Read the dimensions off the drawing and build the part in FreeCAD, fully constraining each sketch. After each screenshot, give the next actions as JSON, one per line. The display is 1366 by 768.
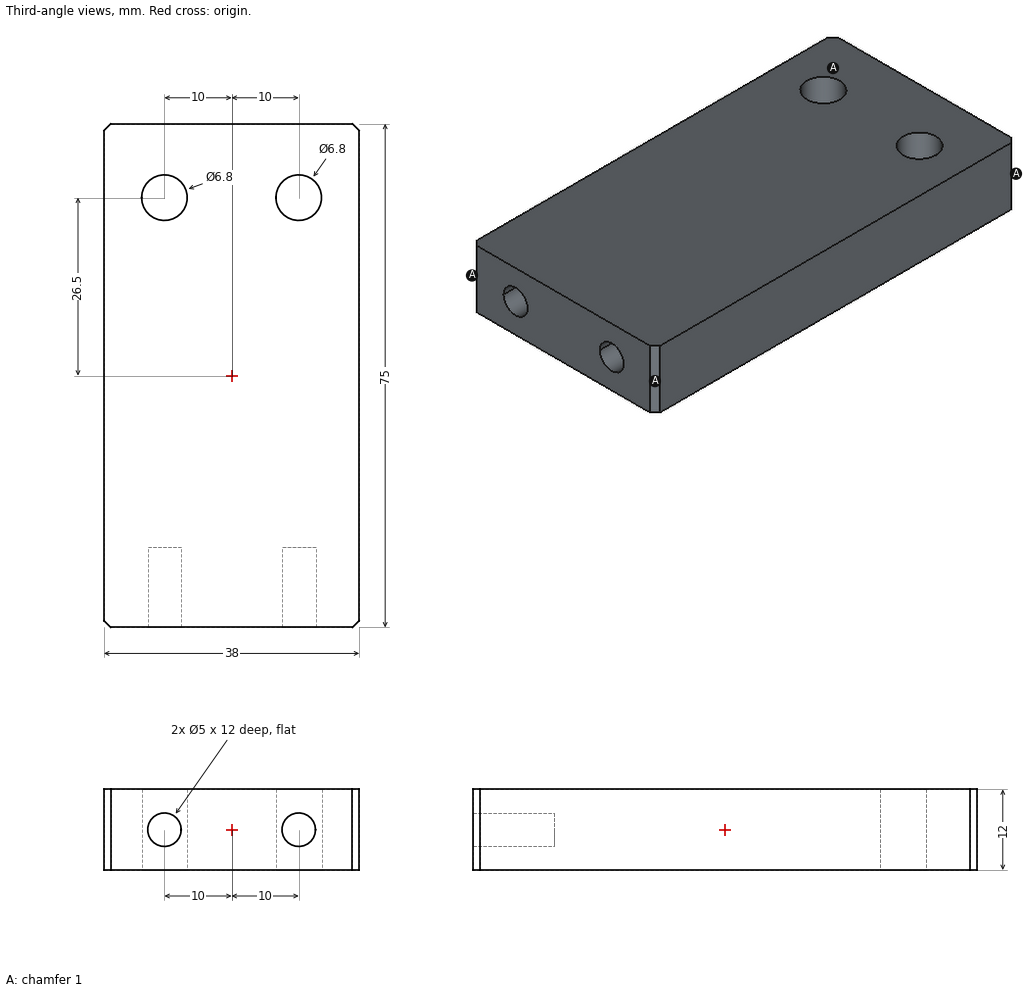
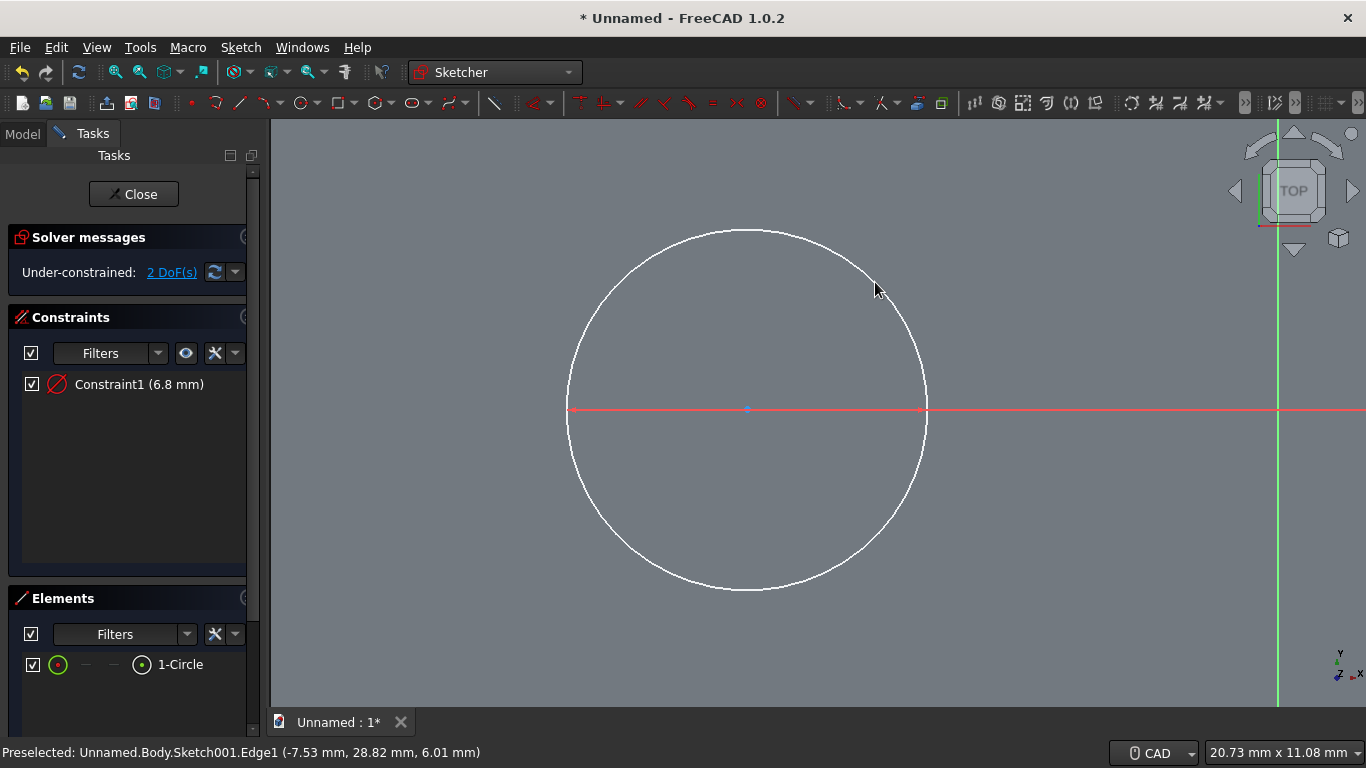
{"action": "key", "text": "d"}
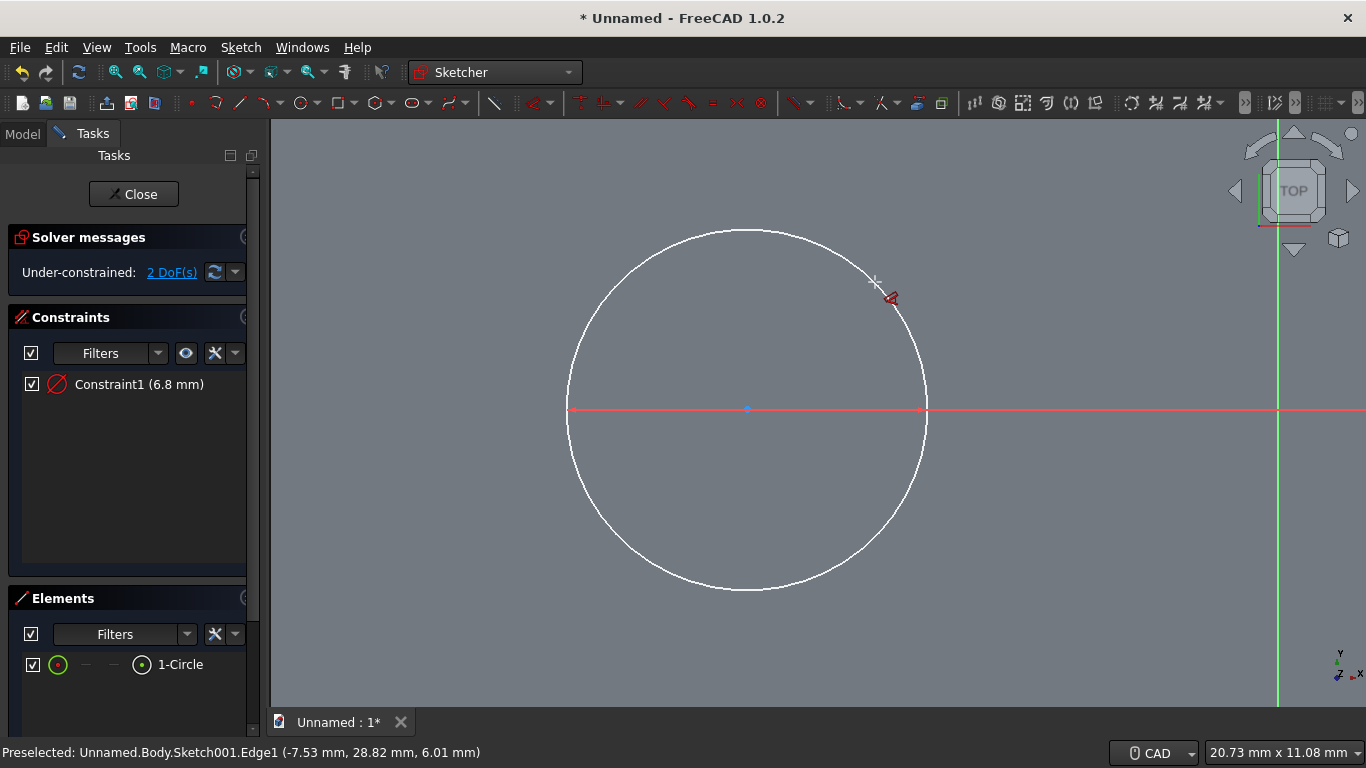
{"action": "left_click", "coordinate": [747, 410]}
{"action": "left_click", "coordinate": [974, 376]}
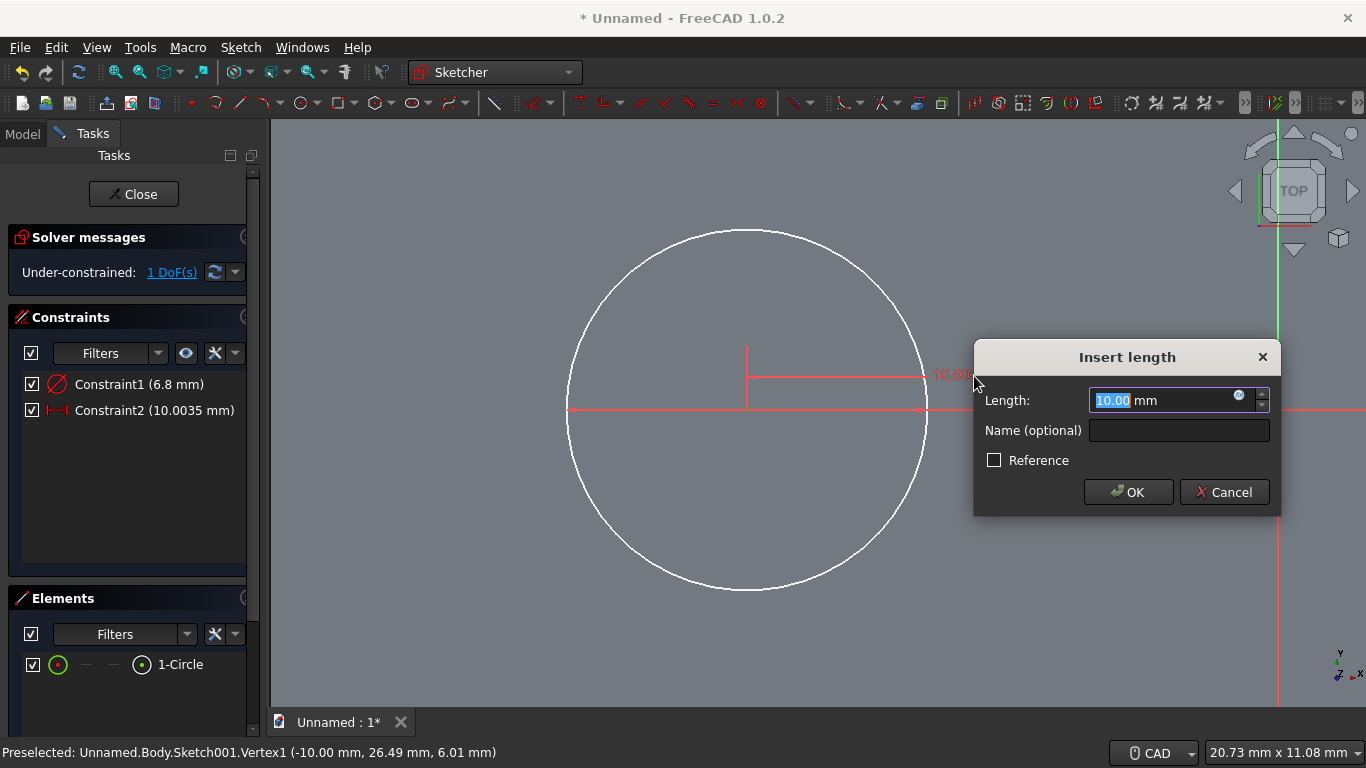
{"action": "type", "text": "10"}
{"action": "key", "text": "Return"}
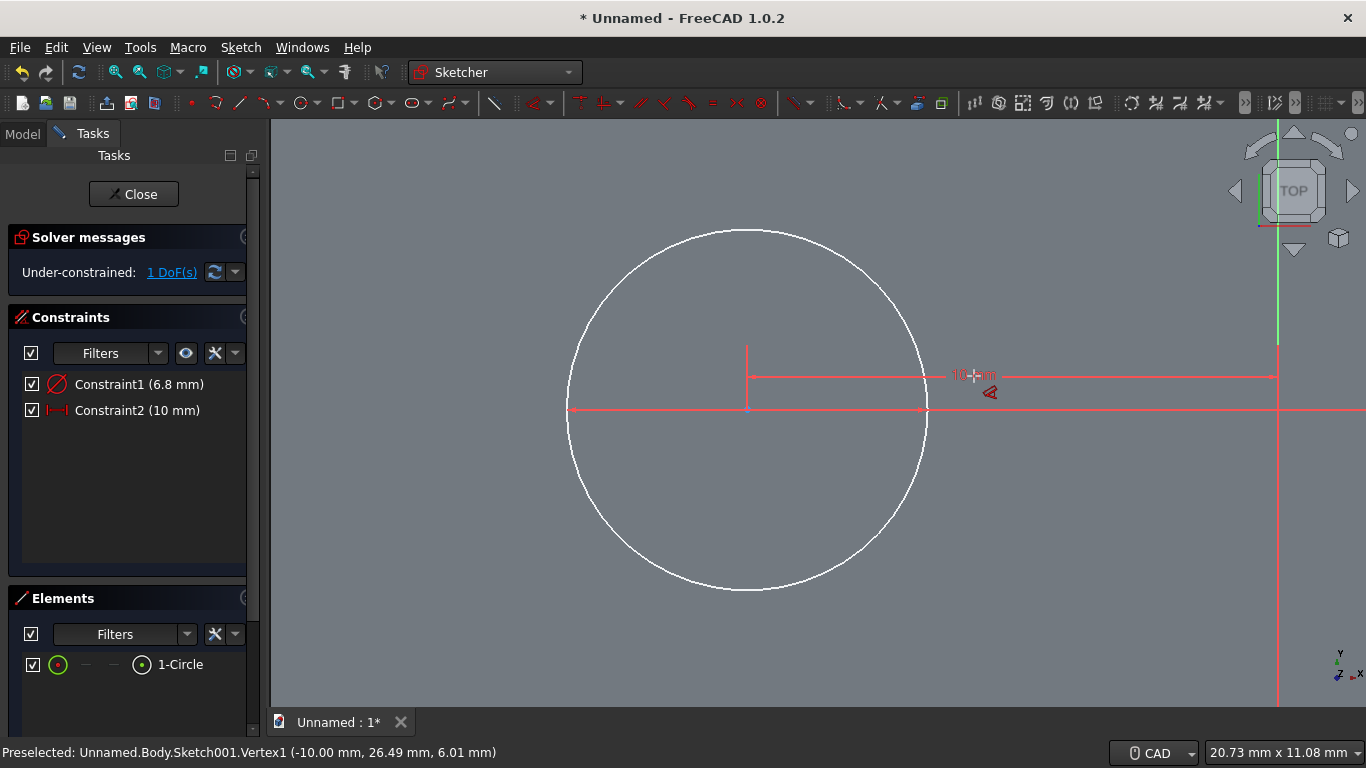
{"action": "left_click", "coordinate": [747, 410]}
{"action": "left_click", "coordinate": [713, 545]}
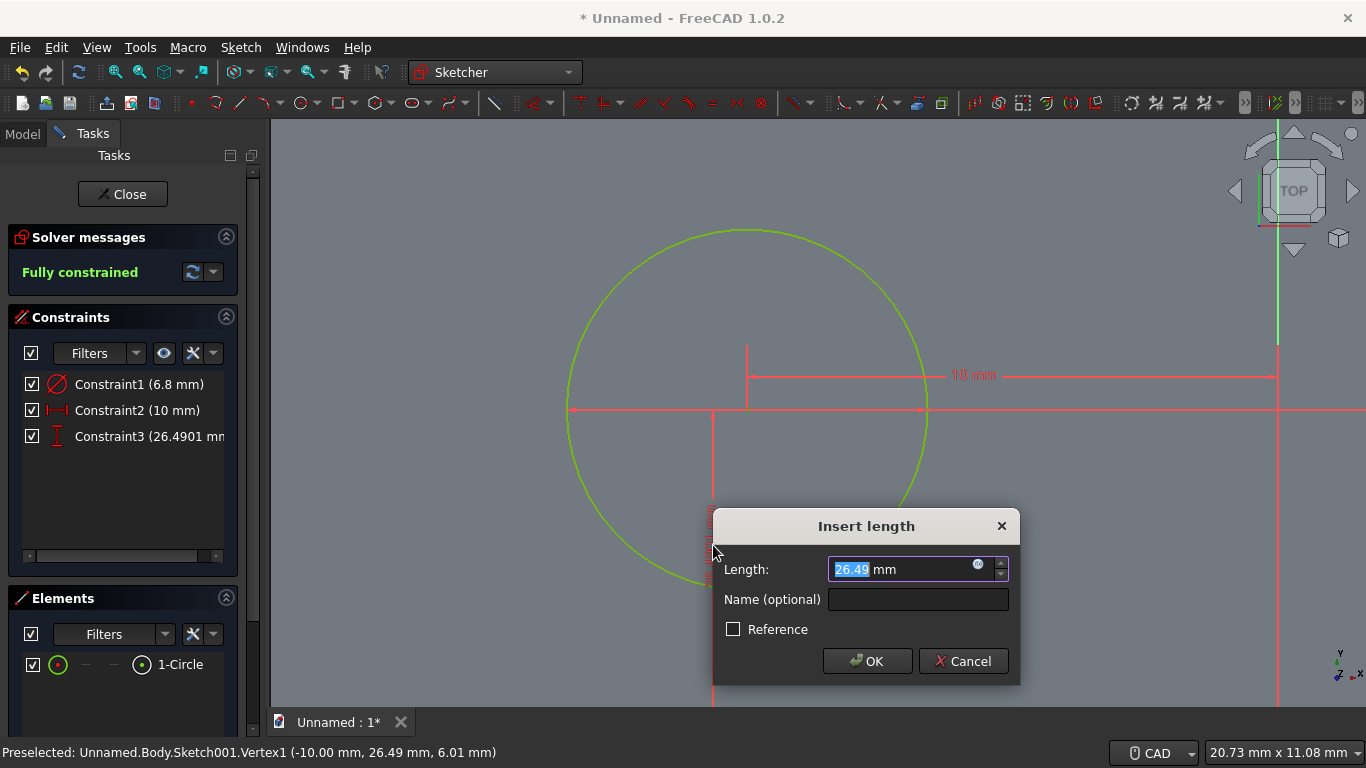
{"action": "type", "text": "26.5"}
{"action": "key", "text": "Return"}
{"action": "key", "text": "Escape"}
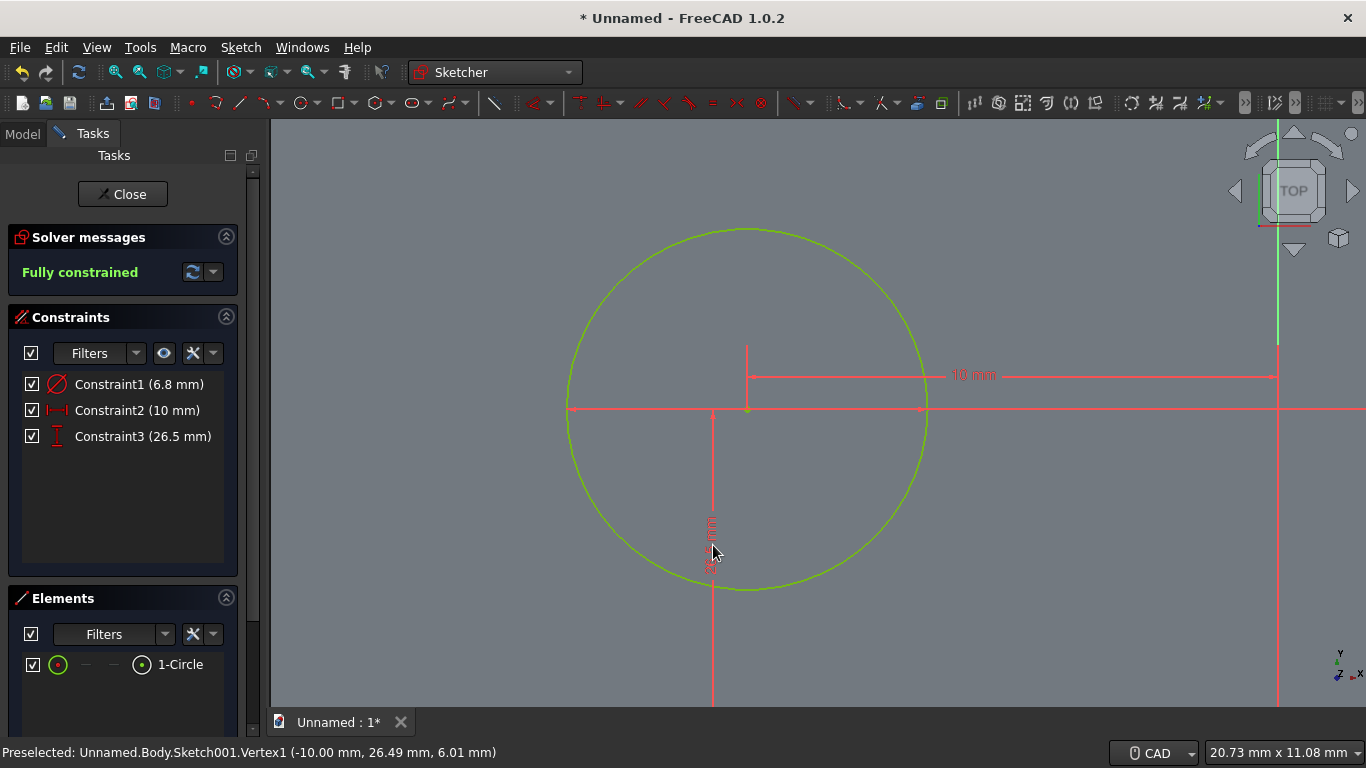
{"action": "left_click", "coordinate": [123, 194]}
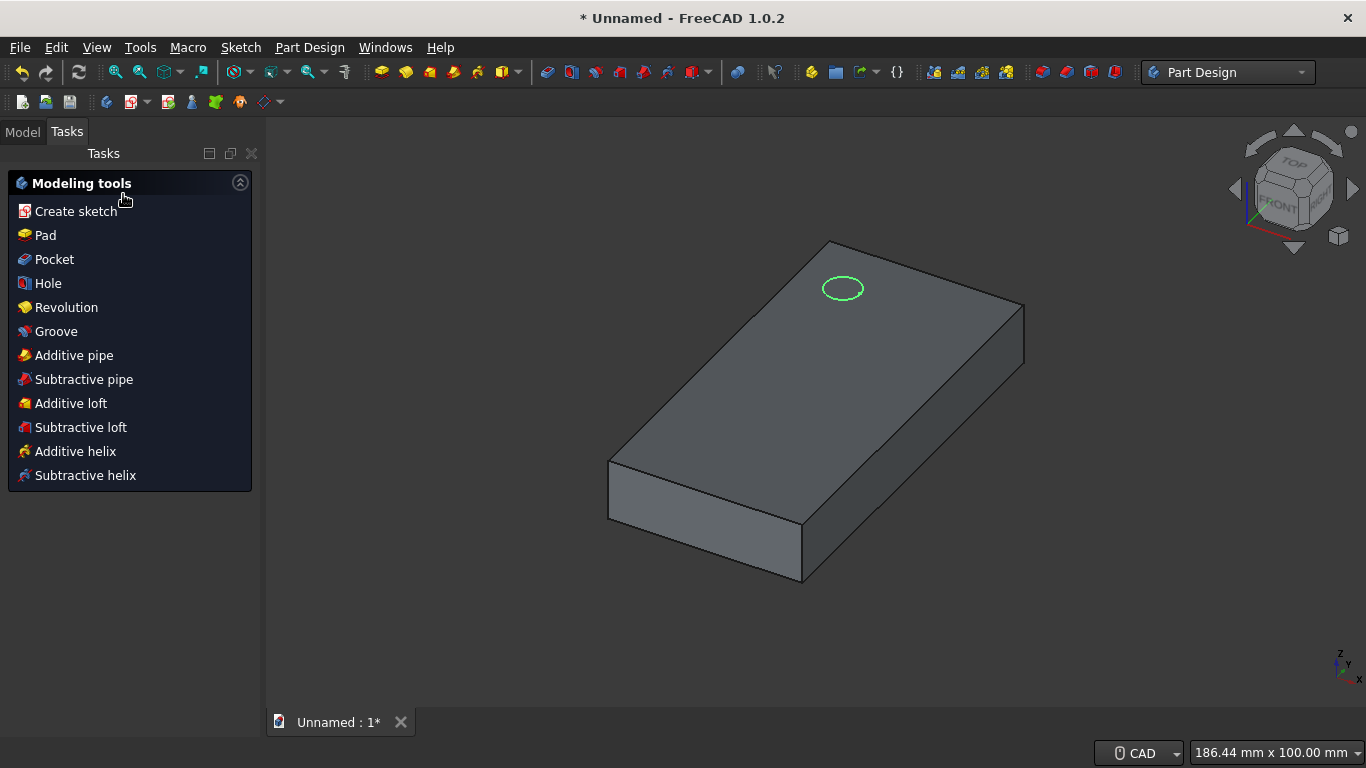
{"action": "left_click", "coordinate": [548, 72]}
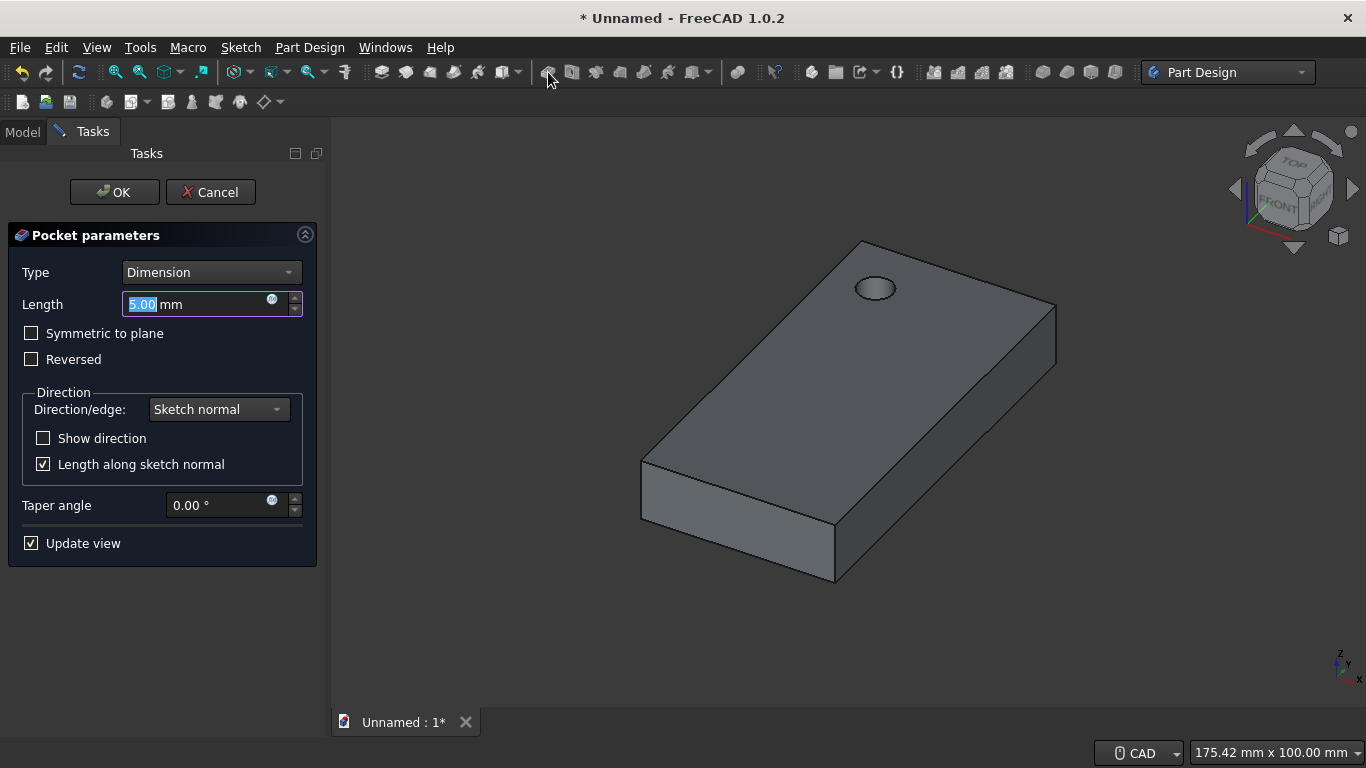
{"action": "left_click", "coordinate": [212, 272]}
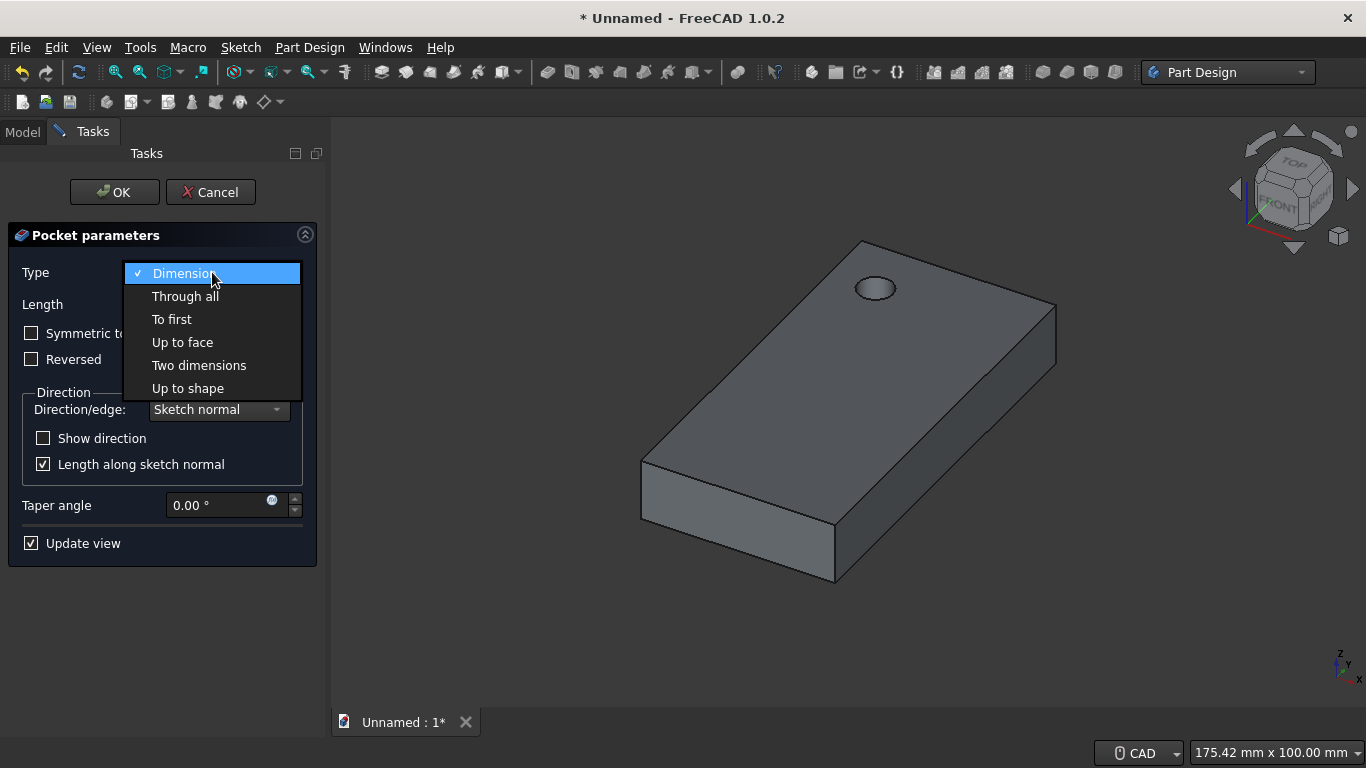
{"action": "left_click", "coordinate": [212, 296]}